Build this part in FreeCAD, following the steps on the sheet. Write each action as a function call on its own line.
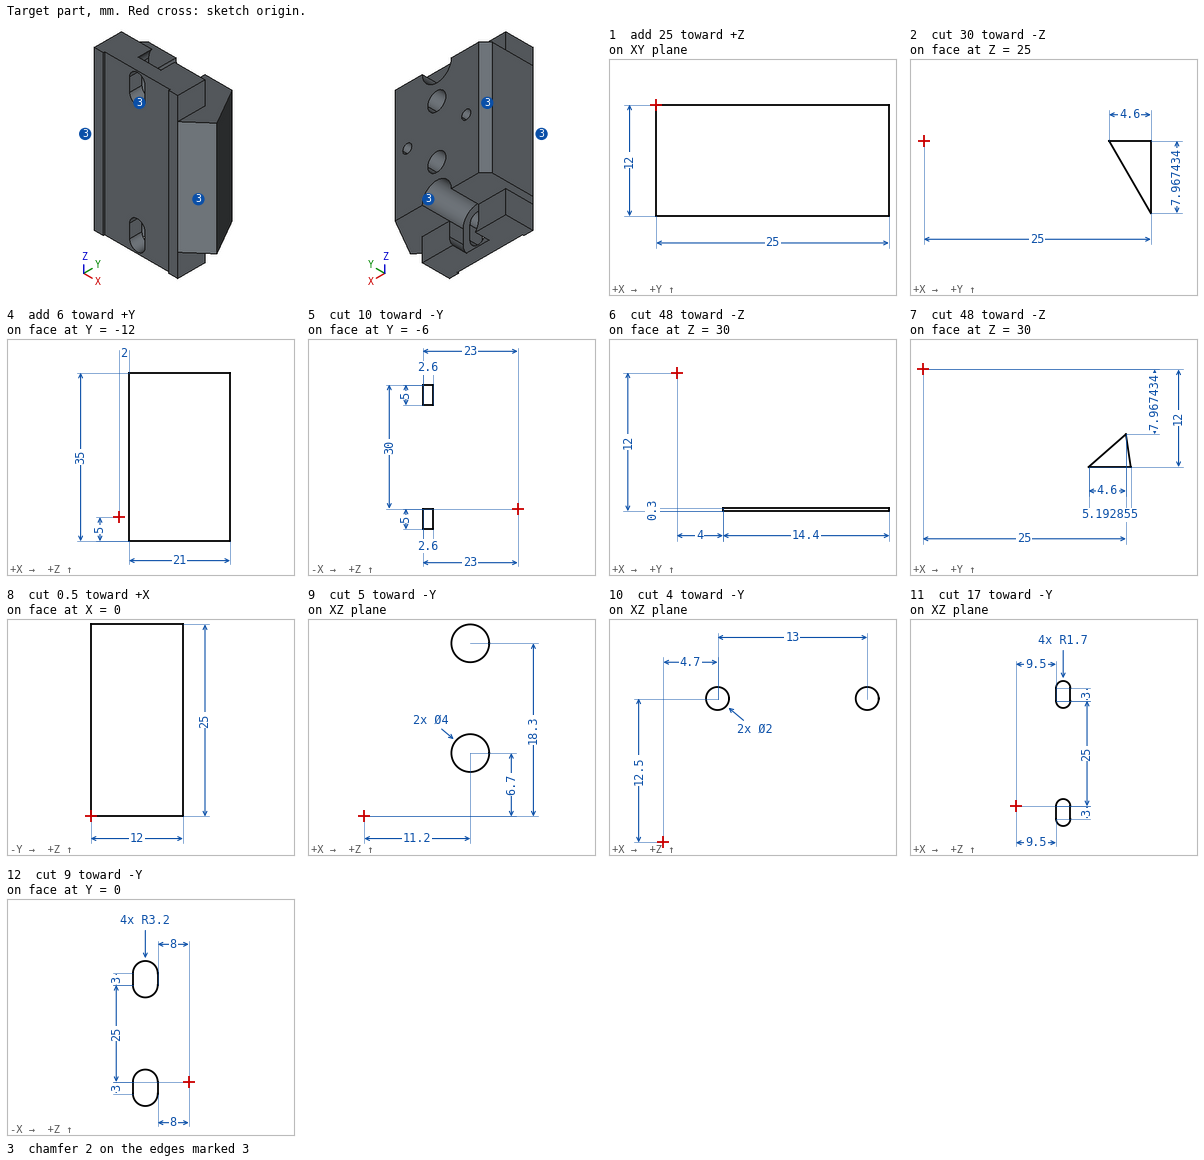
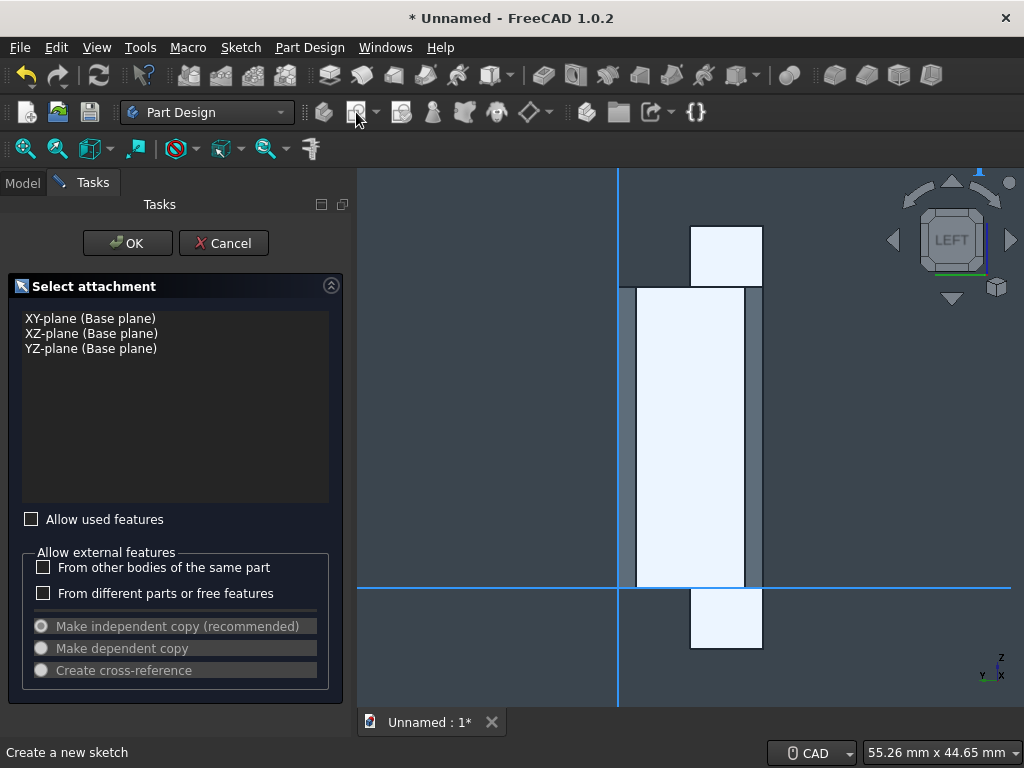
click(82, 334)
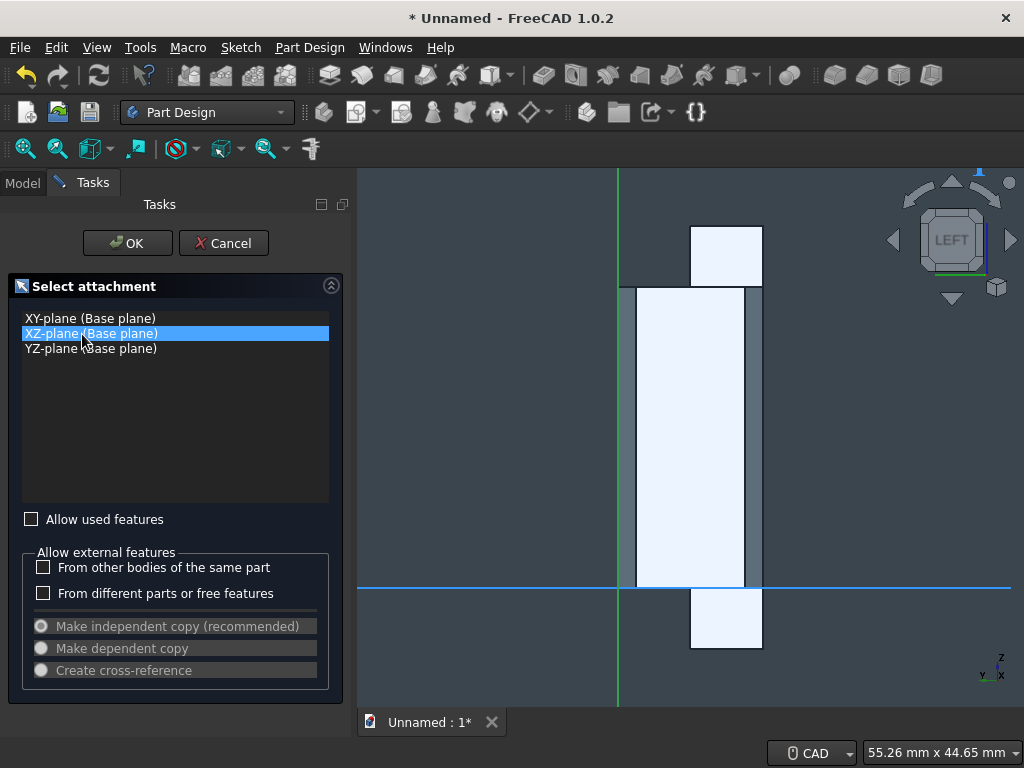
click(128, 243)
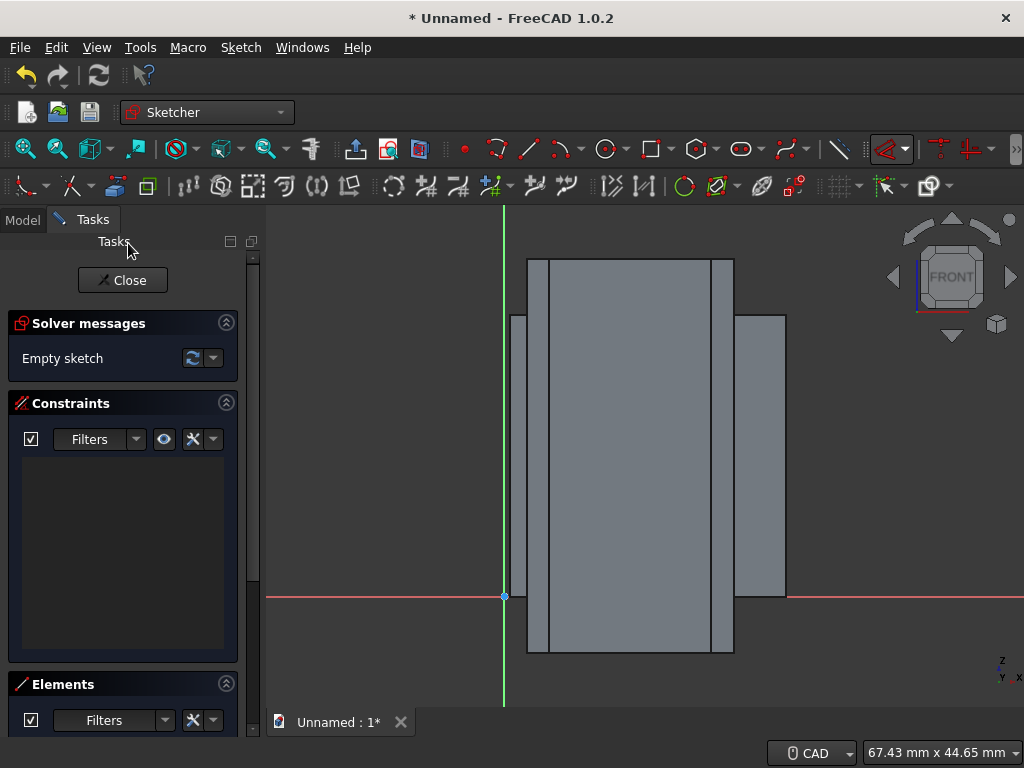
click(420, 150)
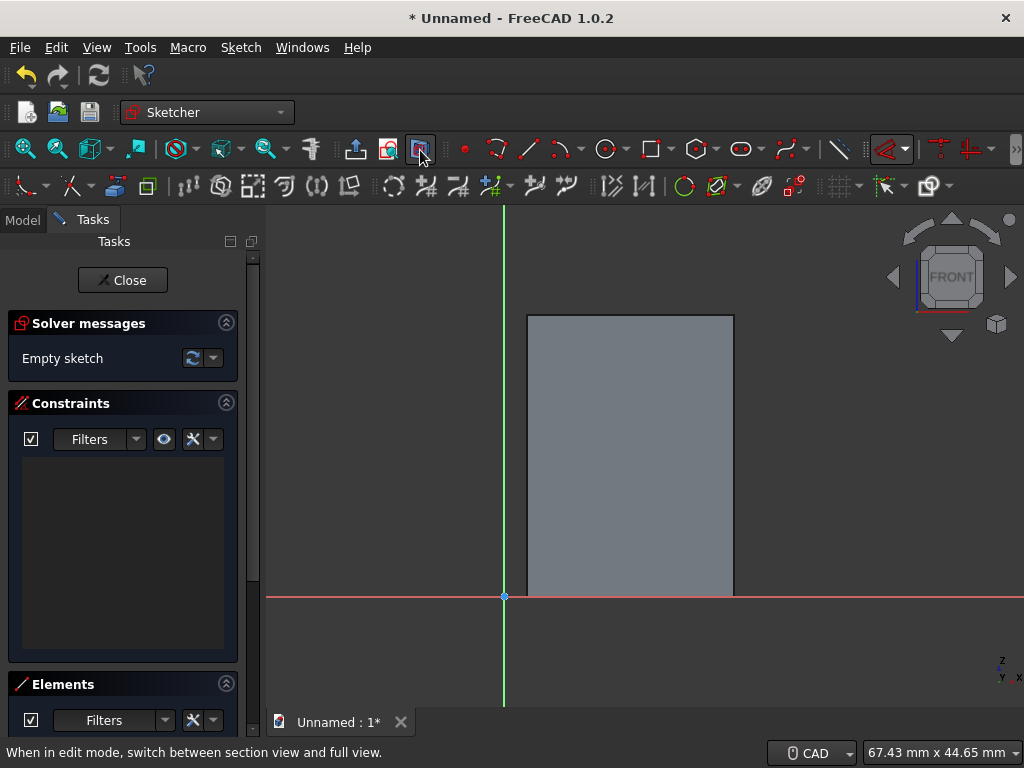
scroll(583, 536, up, 2)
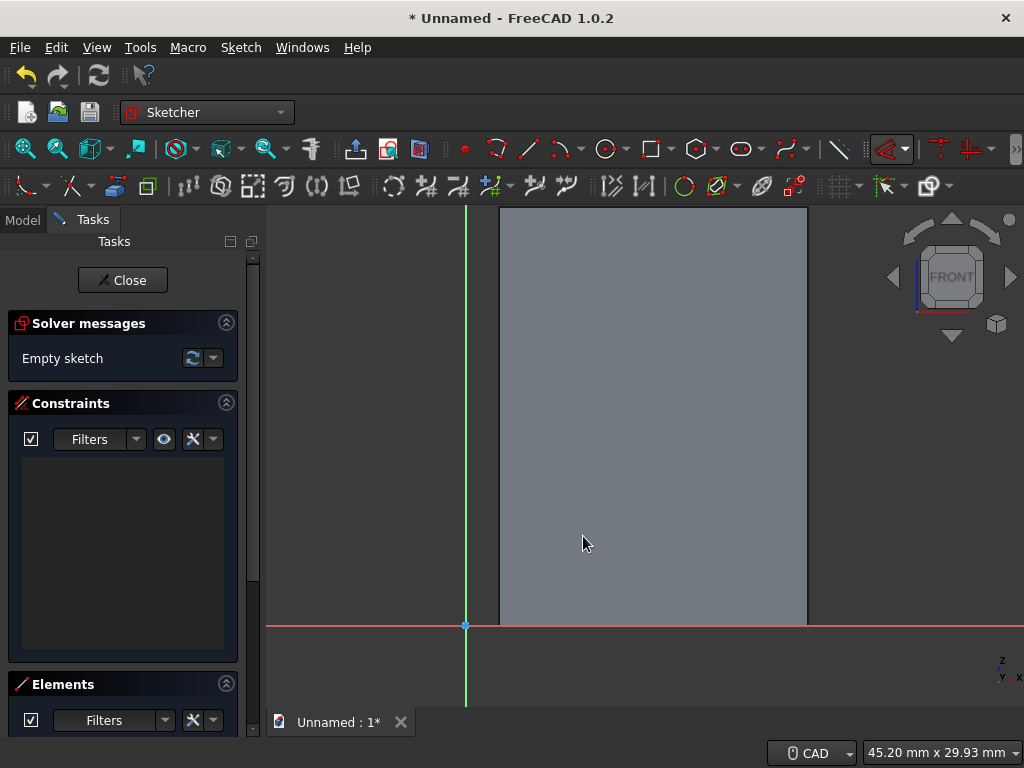
click(606, 150)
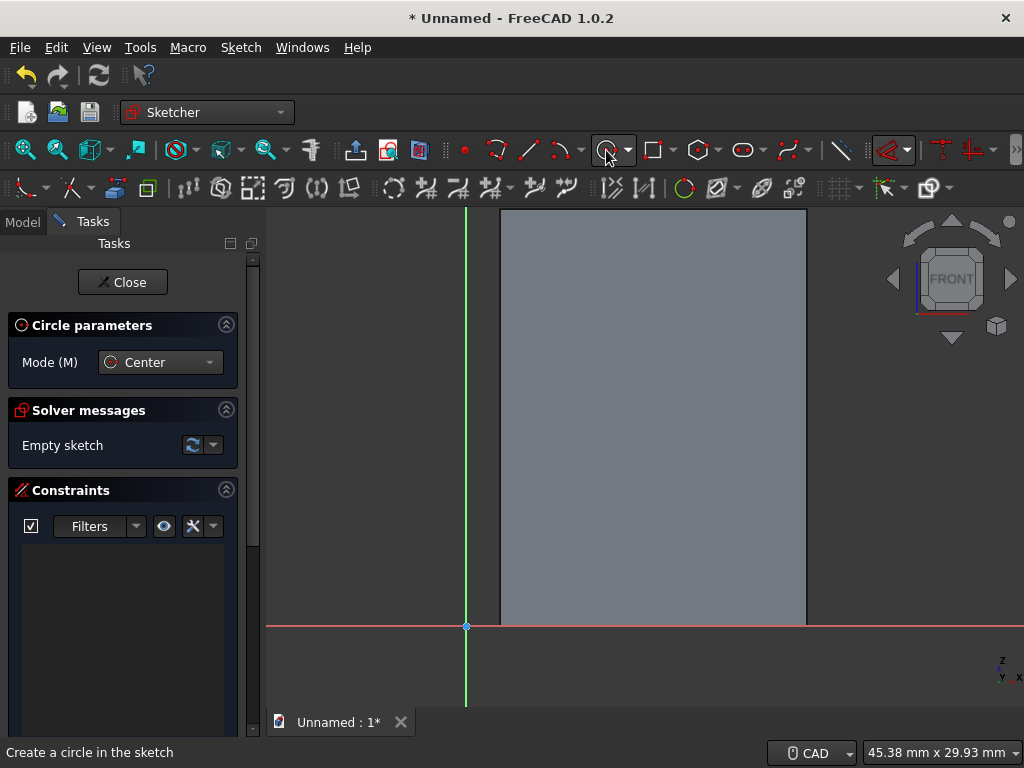
click(653, 514)
click(677, 491)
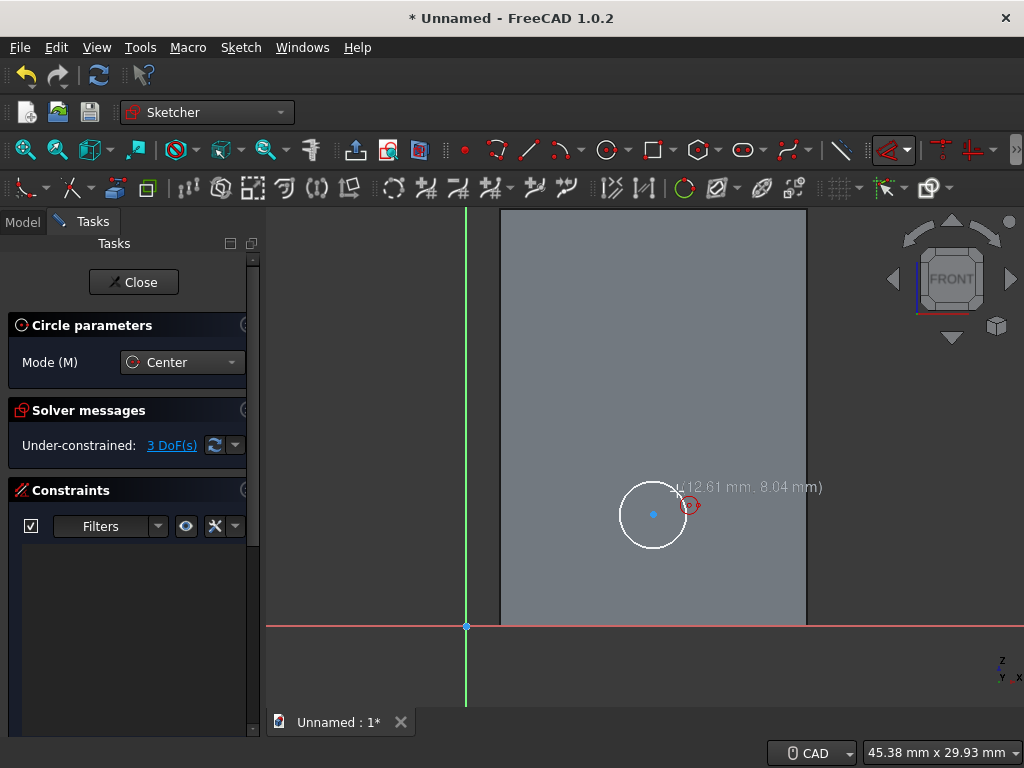
click(653, 321)
click(677, 297)
key(Escape)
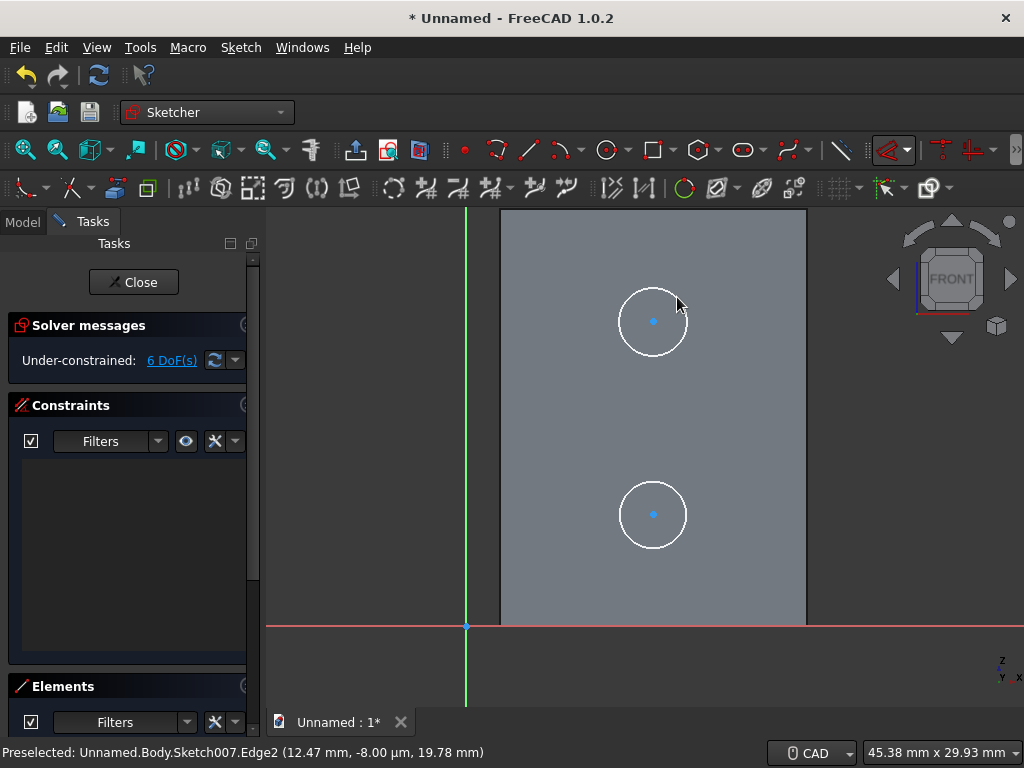
click(676, 491)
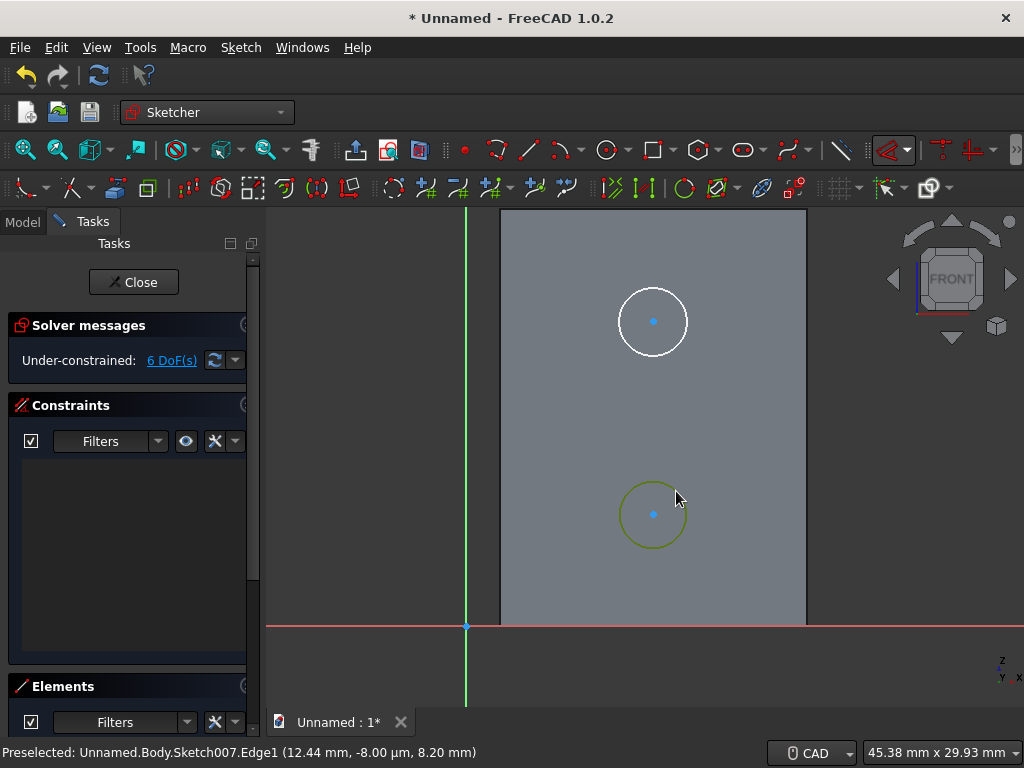
click(677, 298)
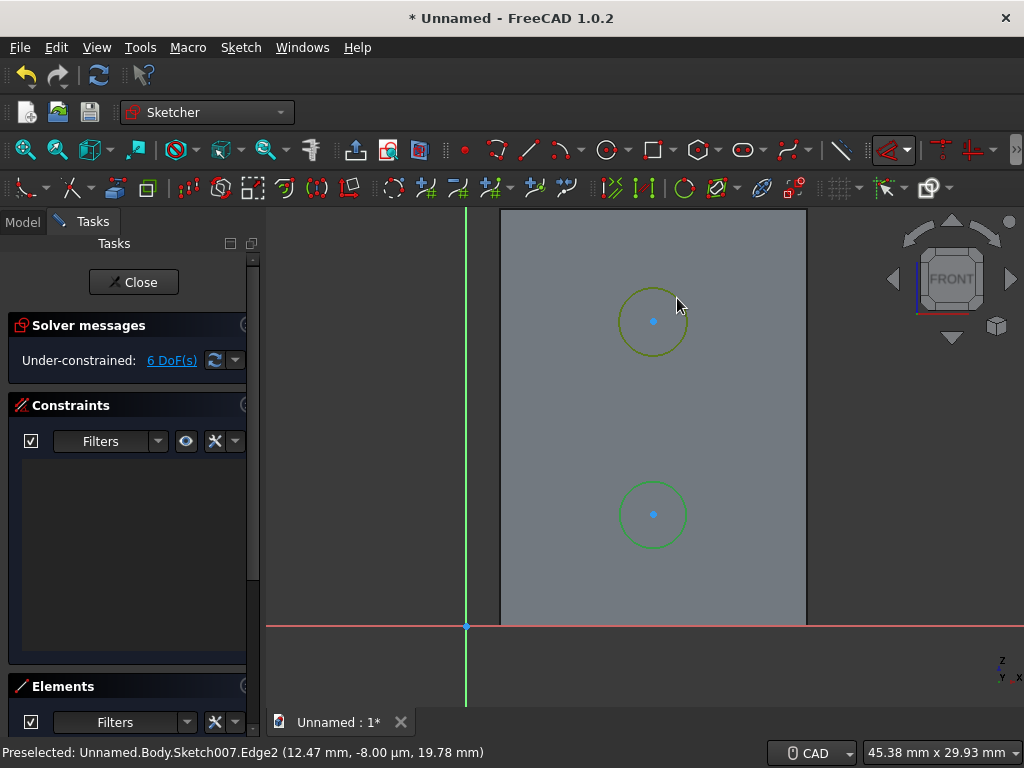
key(e)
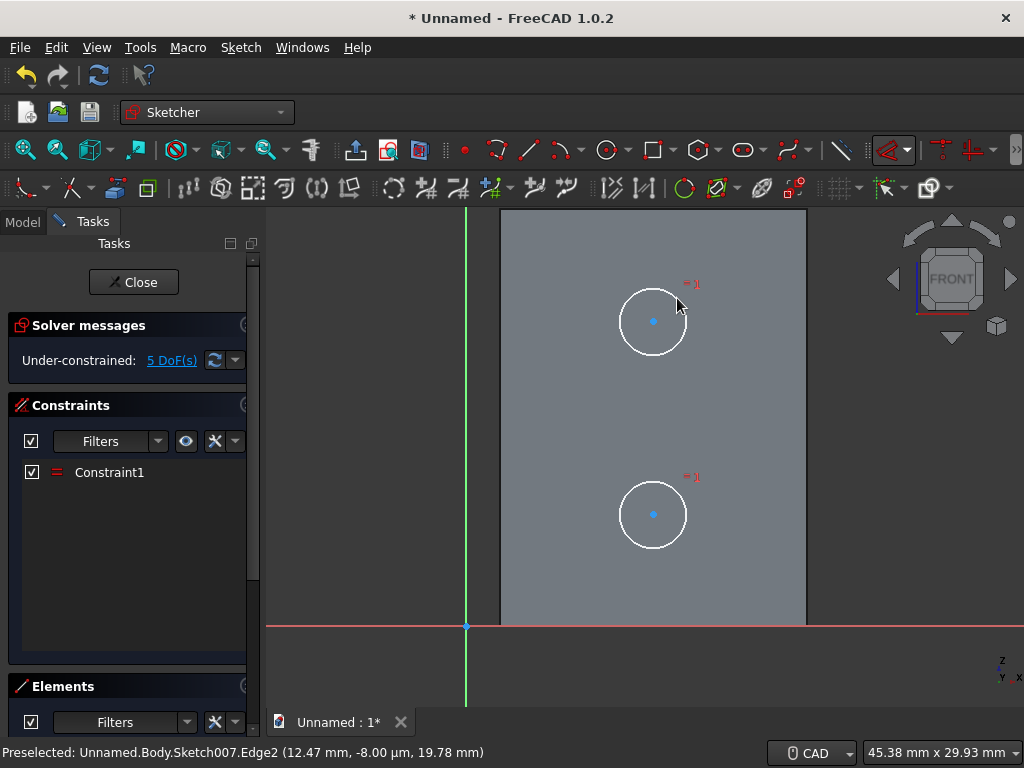
click(653, 515)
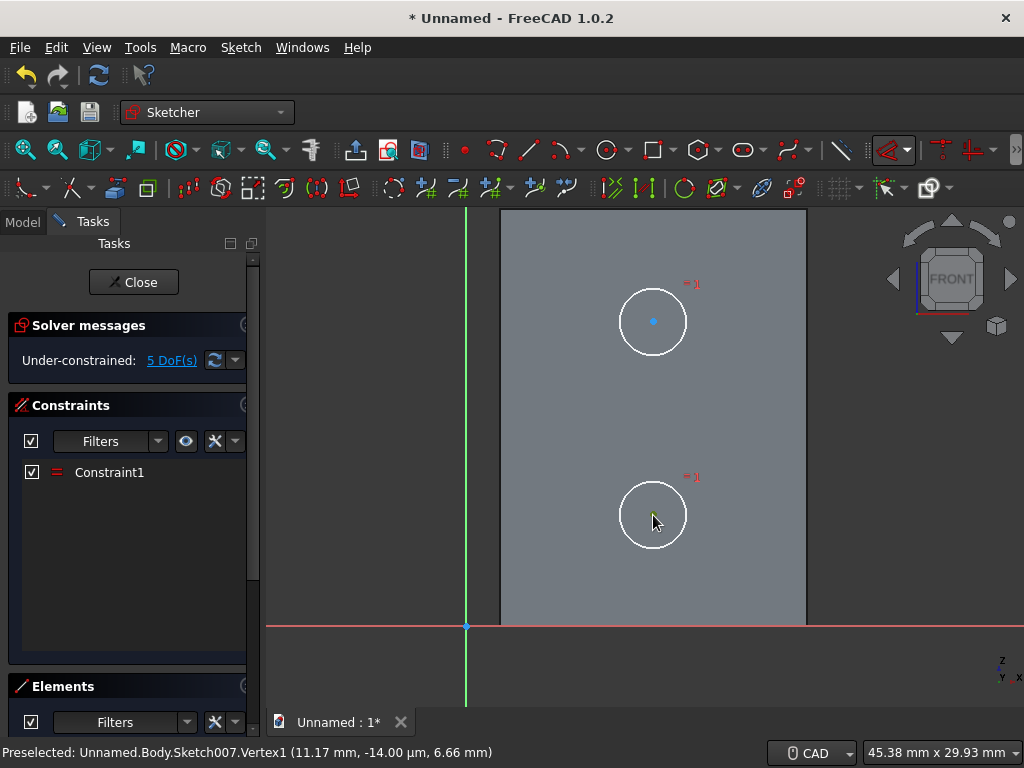
click(653, 322)